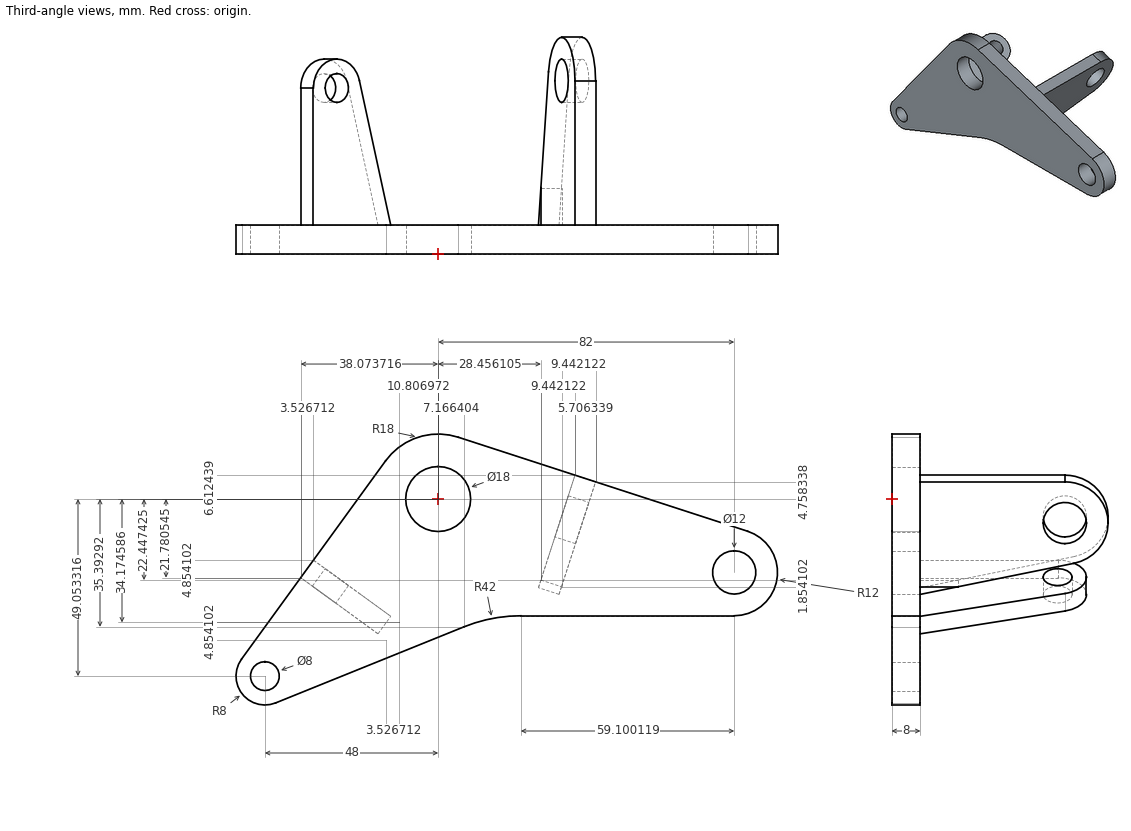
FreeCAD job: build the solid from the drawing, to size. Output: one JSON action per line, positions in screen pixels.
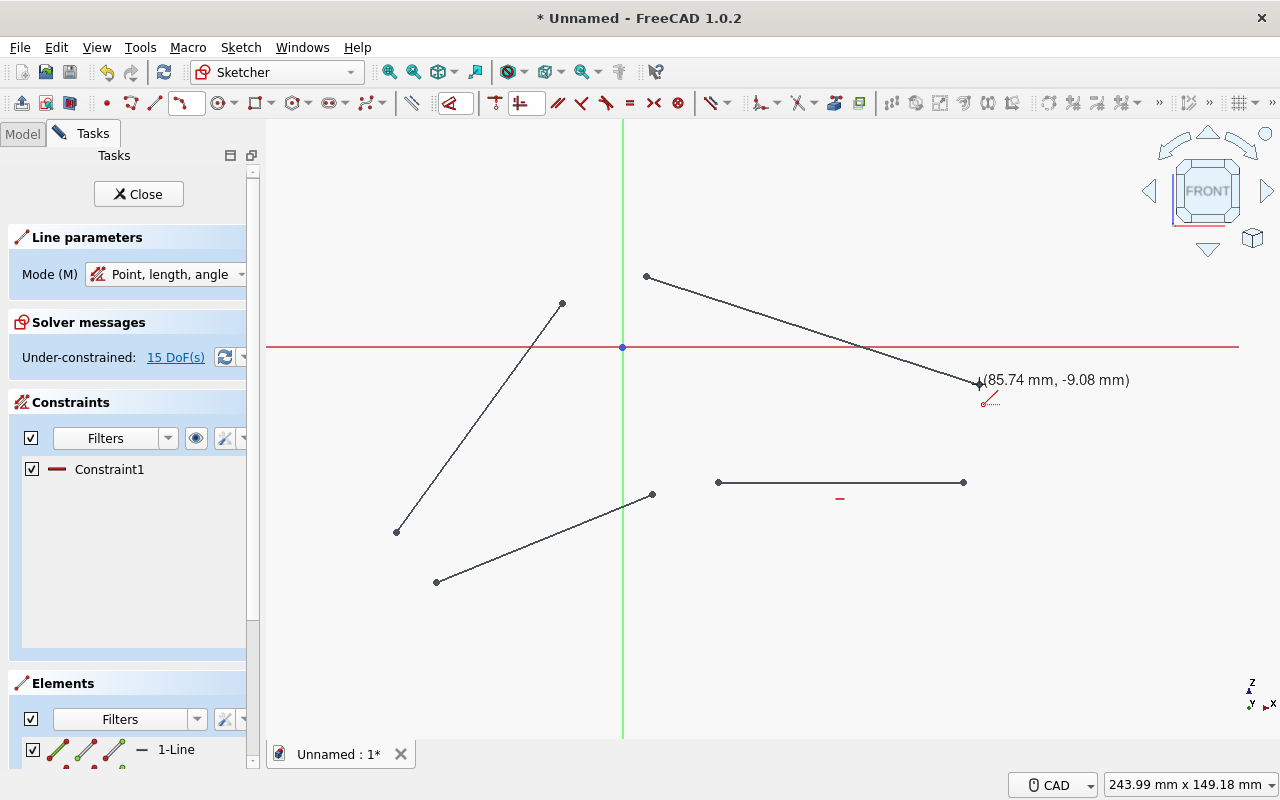
{"action": "key", "text": "g 3 a"}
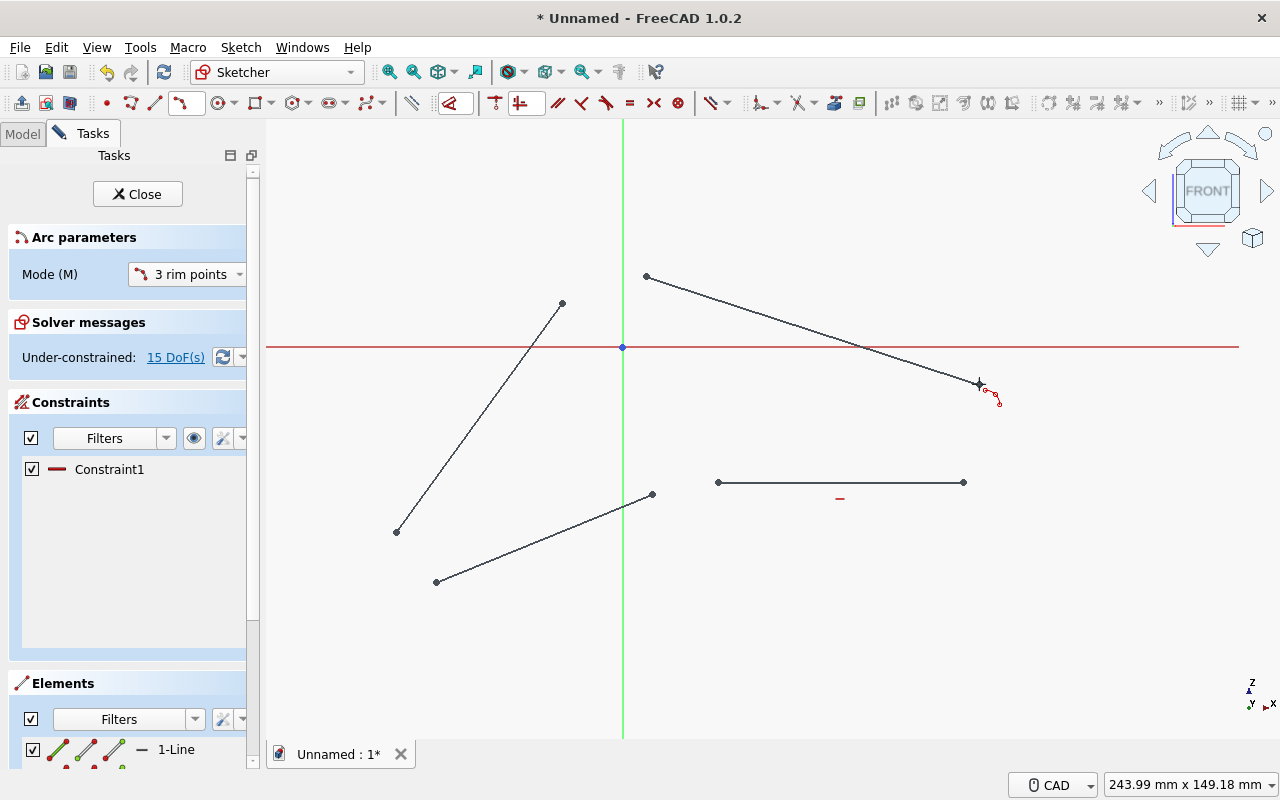
{"action": "left_click", "coordinate": [718, 483]}
{"action": "left_click", "coordinate": [652, 495]}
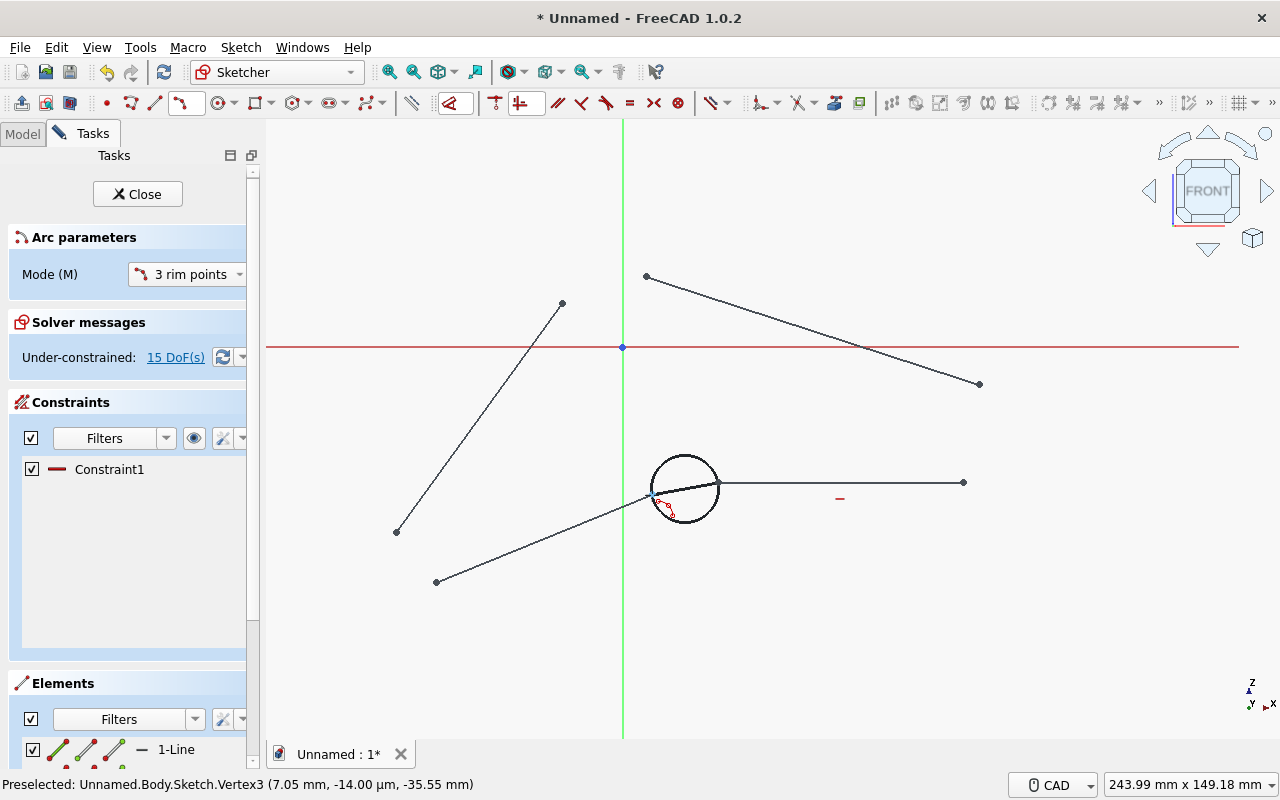
{"action": "scroll", "coordinate": [685, 485], "scroll_direction": "up", "scroll_amount": 8}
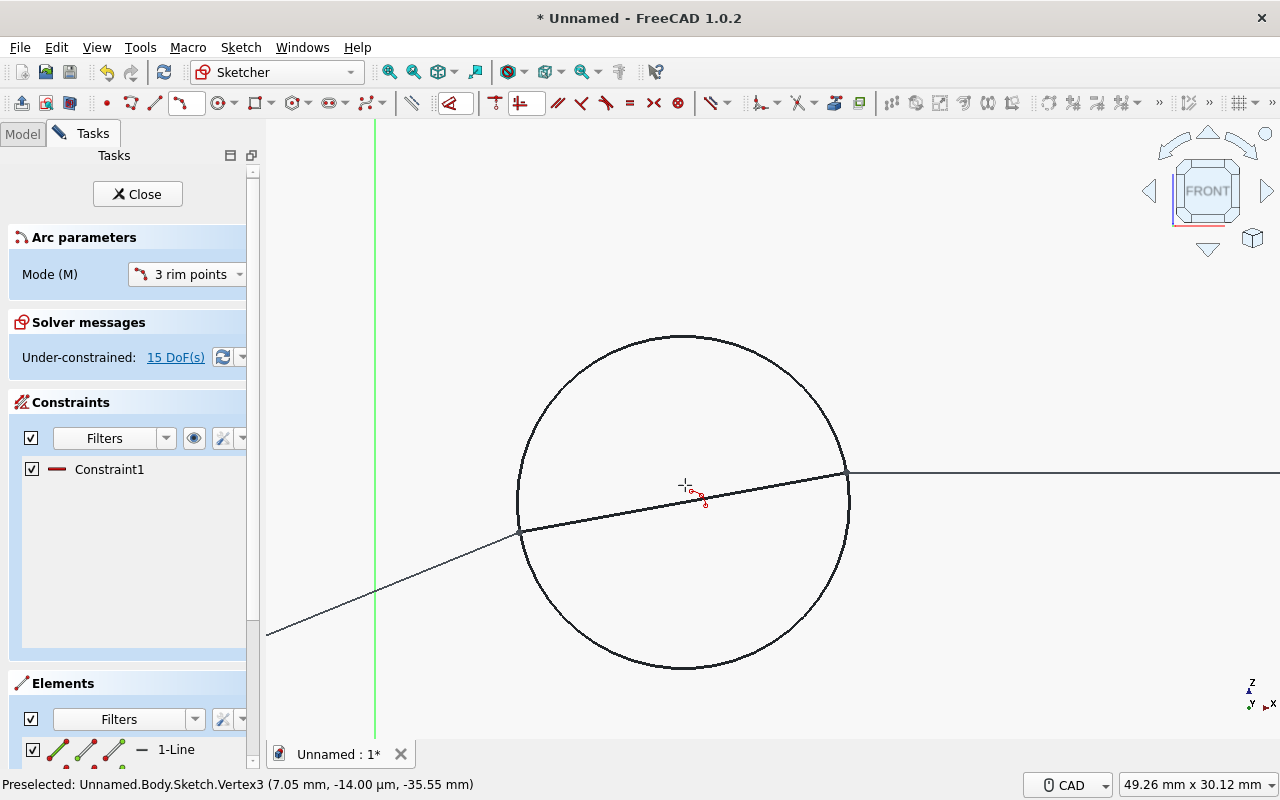
{"action": "left_click", "coordinate": [681, 482]}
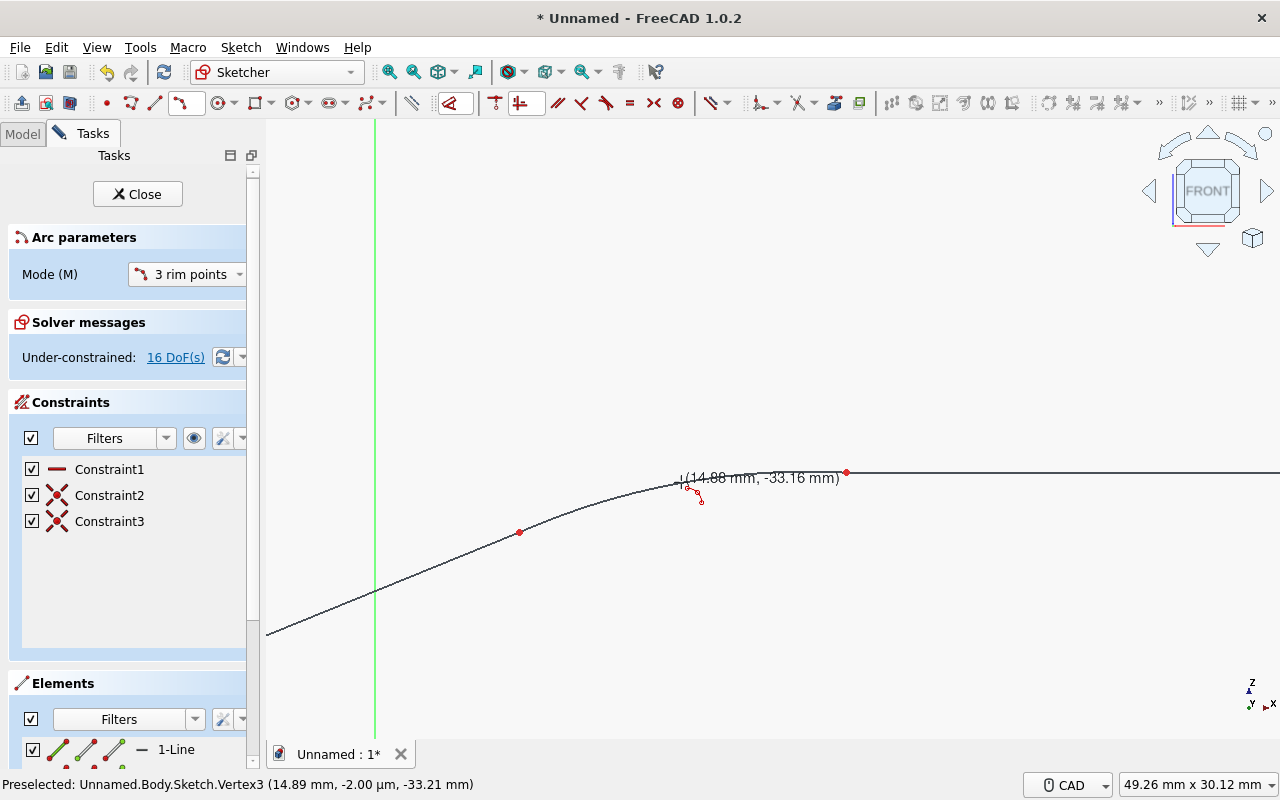
{"action": "scroll", "coordinate": [685, 486], "scroll_direction": "down", "scroll_amount": 8}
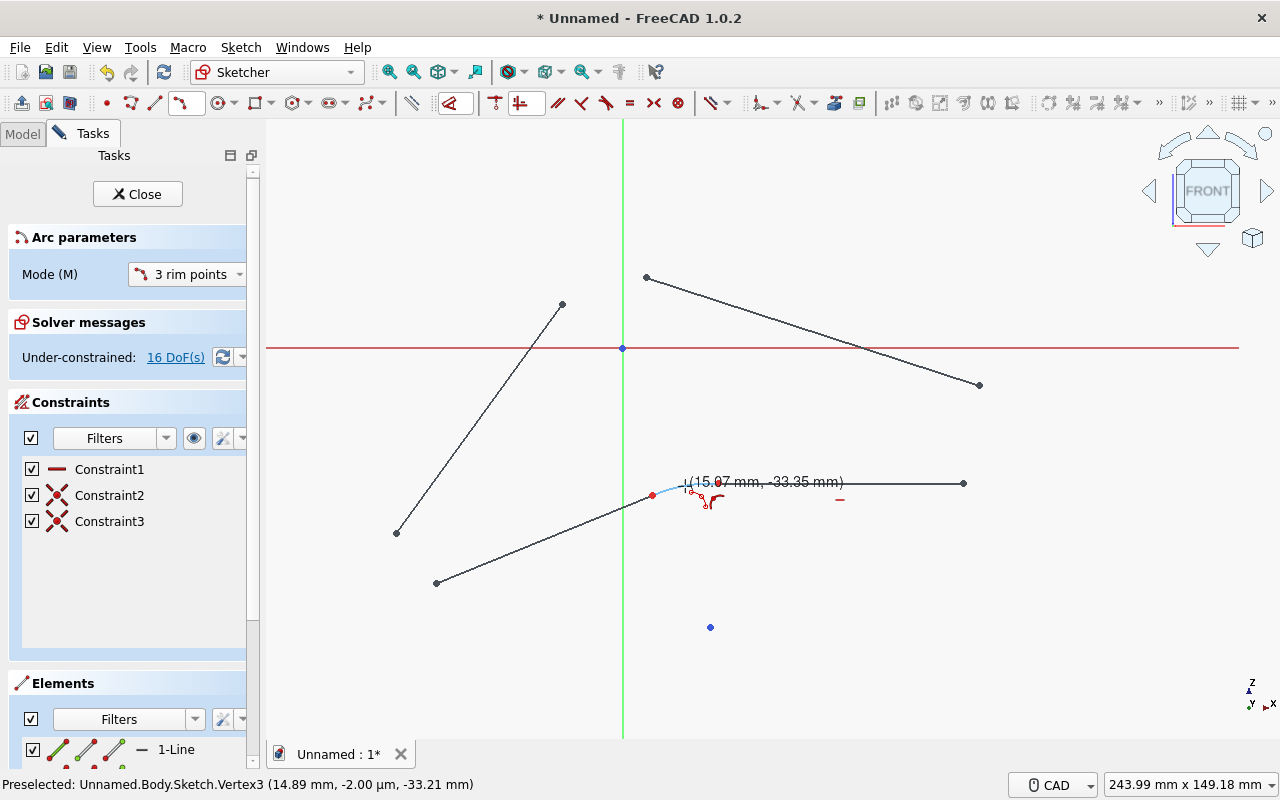
{"action": "left_click", "coordinate": [436, 584]}
{"action": "left_click", "coordinate": [396, 534]}
{"action": "left_click", "coordinate": [397, 572]}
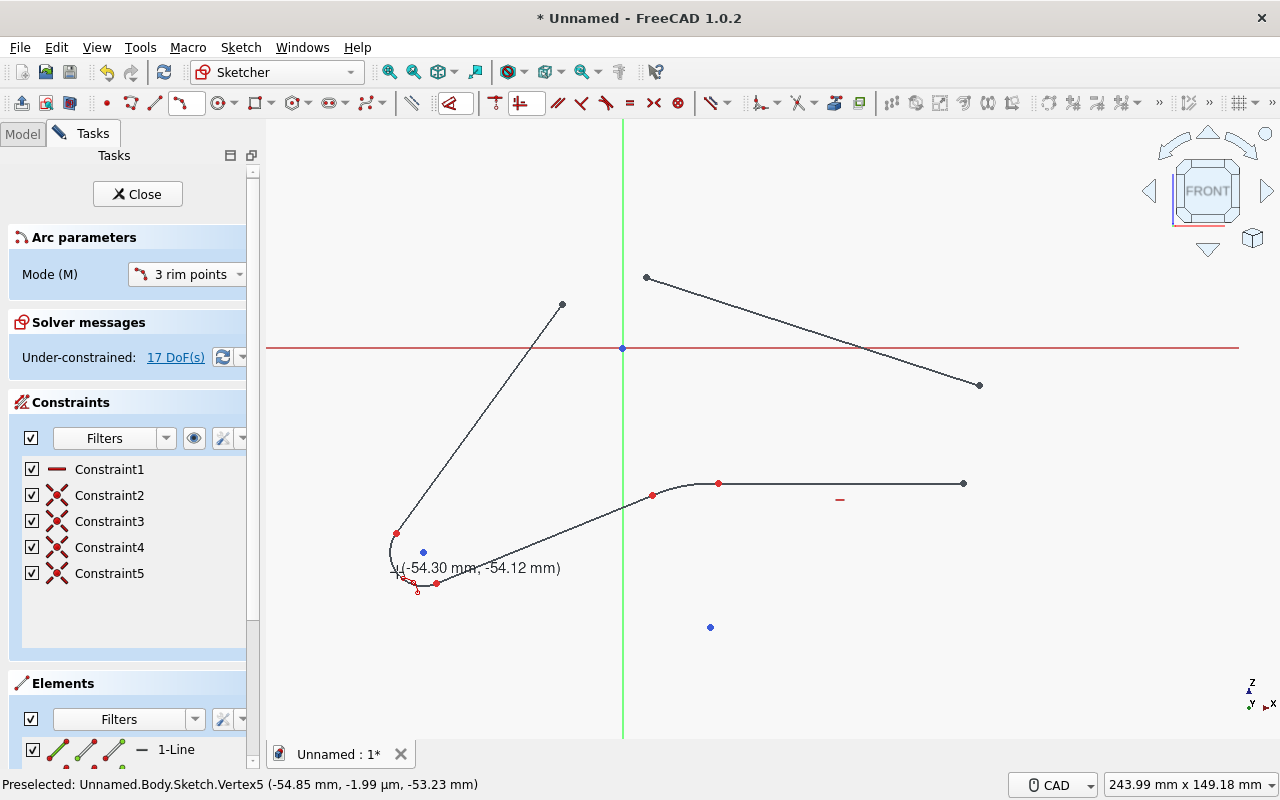
{"action": "left_click", "coordinate": [562, 305]}
{"action": "left_click", "coordinate": [646, 278]}
{"action": "left_click", "coordinate": [600, 277]}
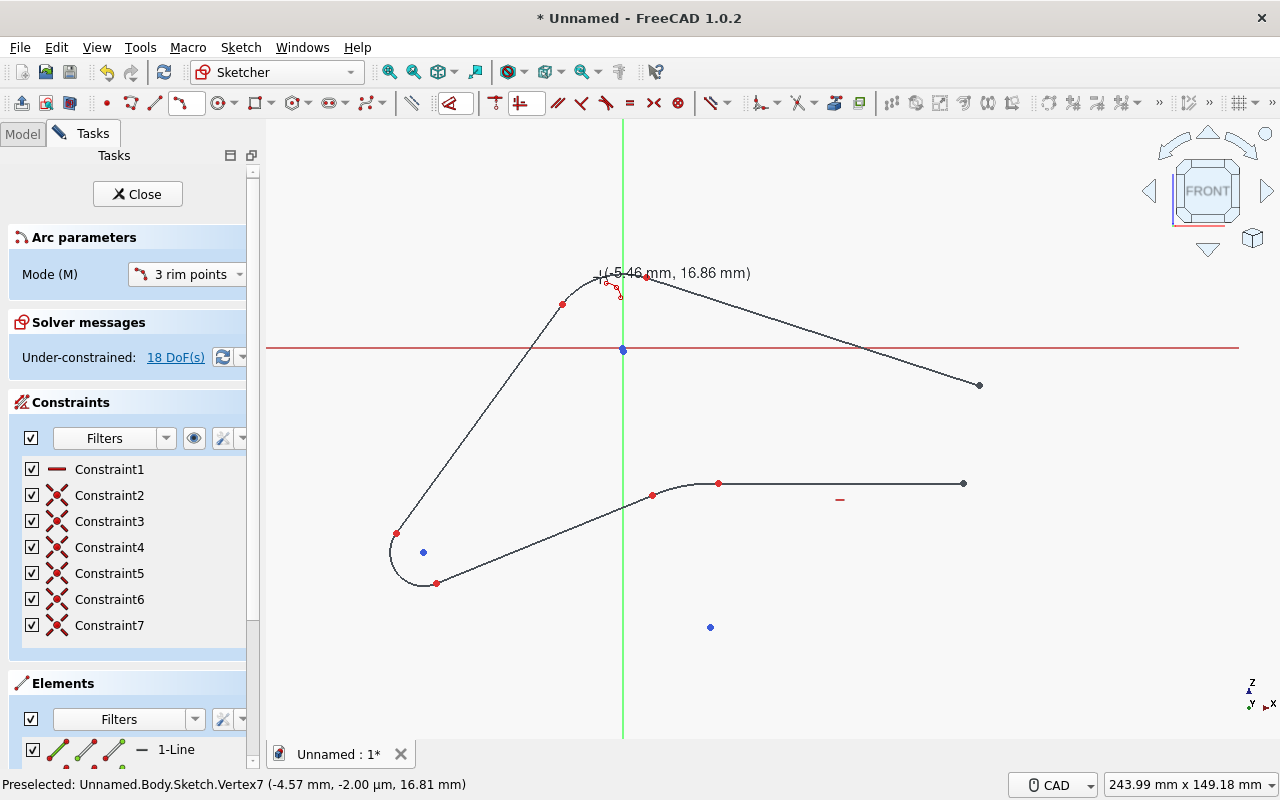
{"action": "left_click", "coordinate": [979, 386]}
{"action": "left_click", "coordinate": [963, 484]}
{"action": "left_click", "coordinate": [1013, 440]}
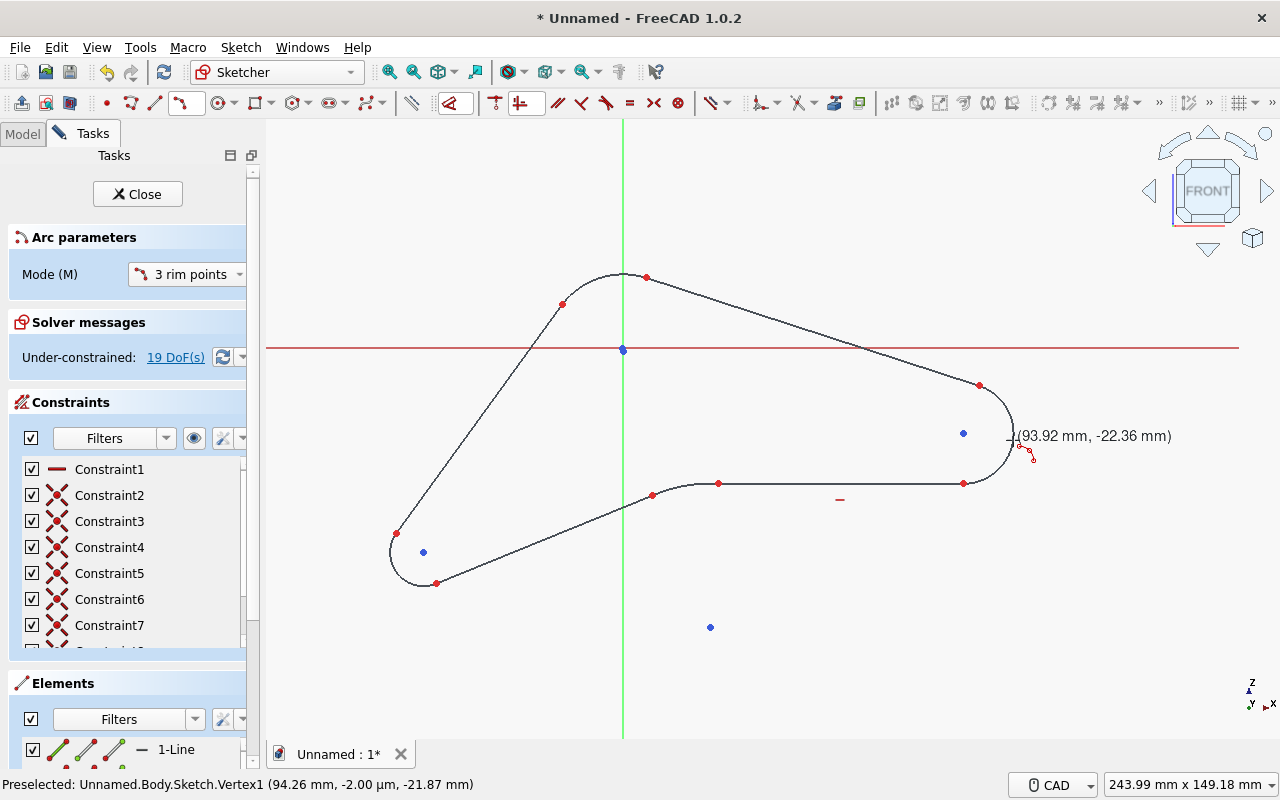
{"action": "left_click", "coordinate": [218, 104]}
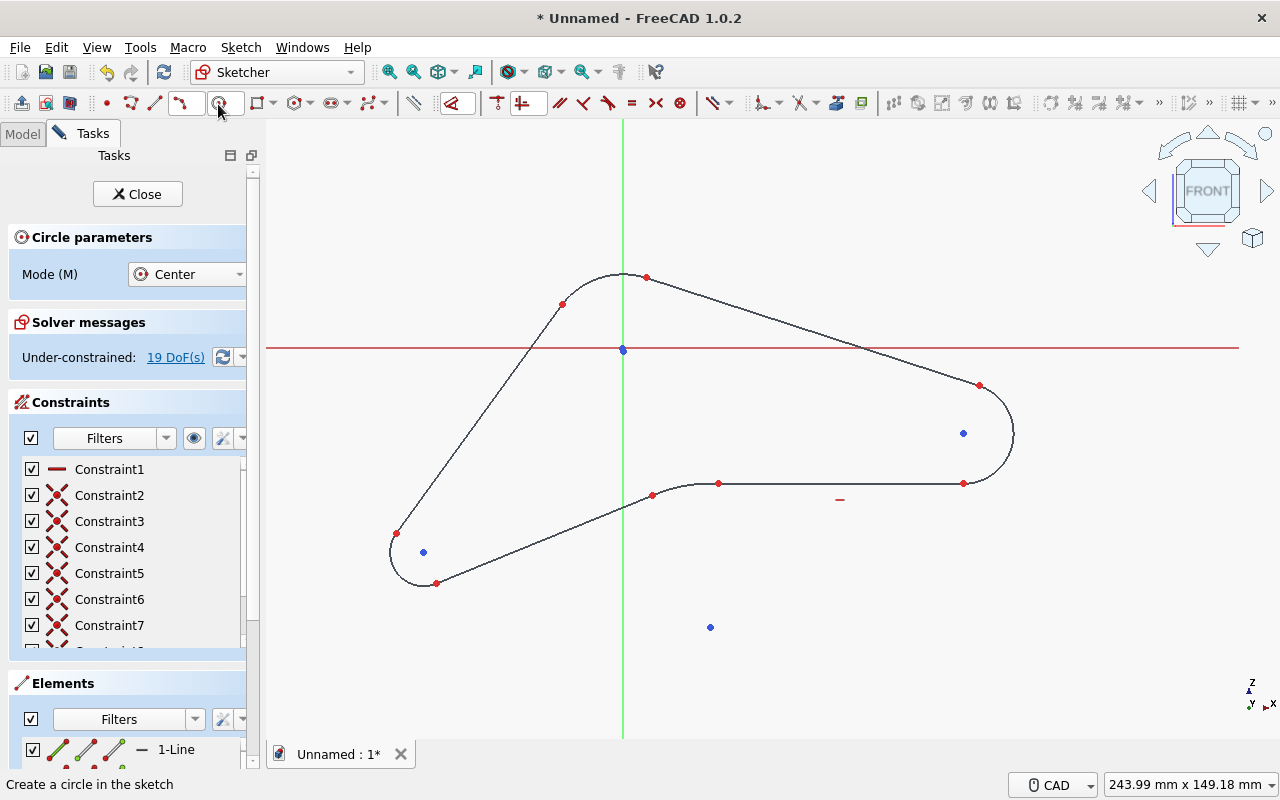
{"action": "left_click", "coordinate": [623, 348]}
{"action": "mouse_move", "coordinate": [649, 322]}